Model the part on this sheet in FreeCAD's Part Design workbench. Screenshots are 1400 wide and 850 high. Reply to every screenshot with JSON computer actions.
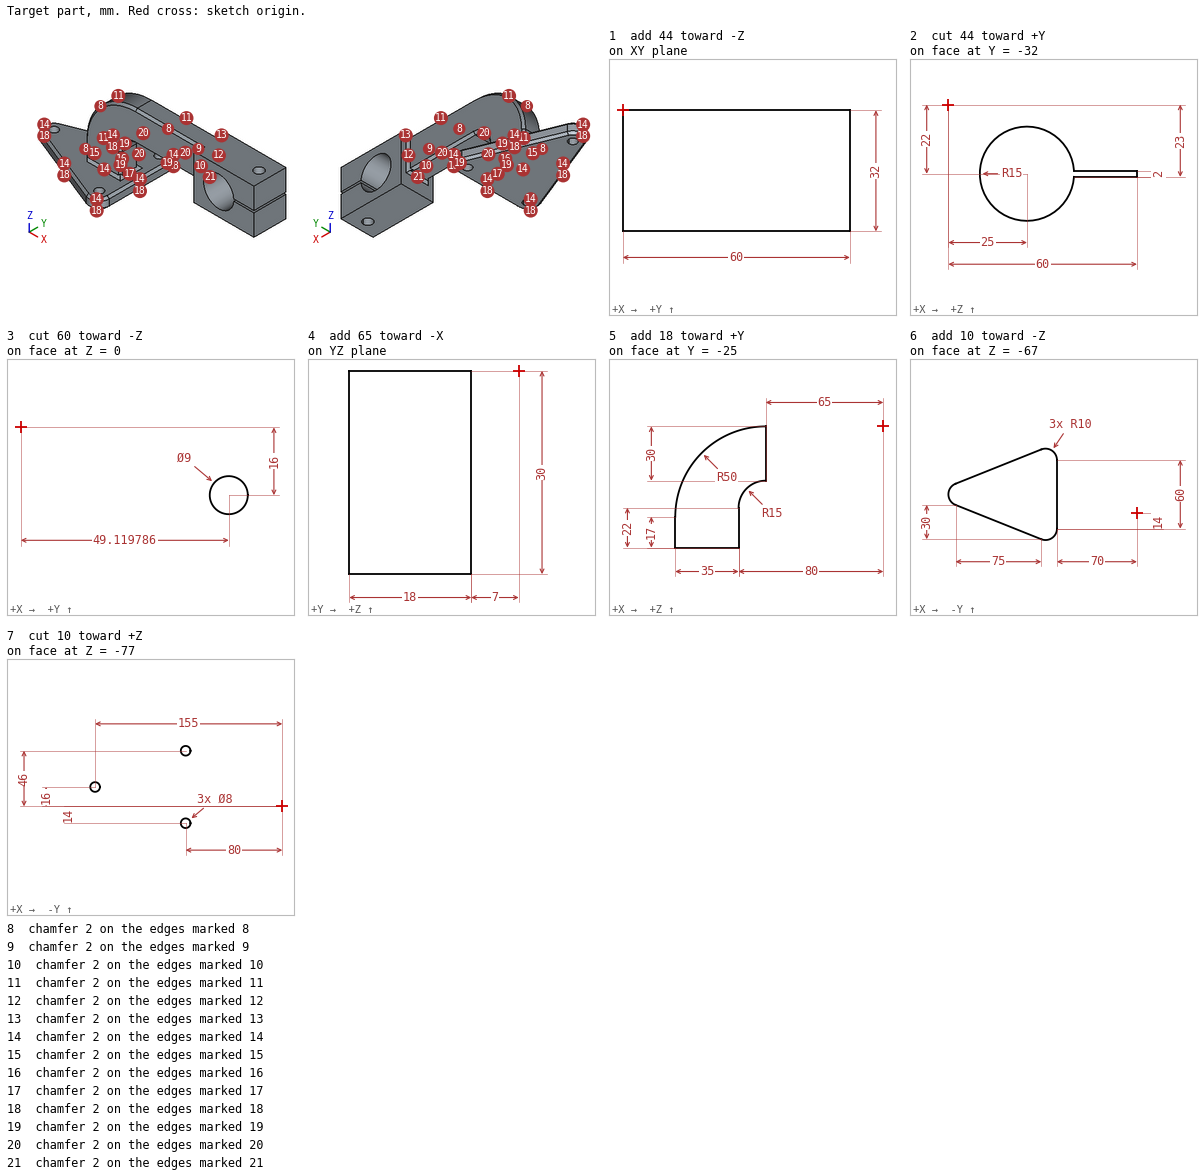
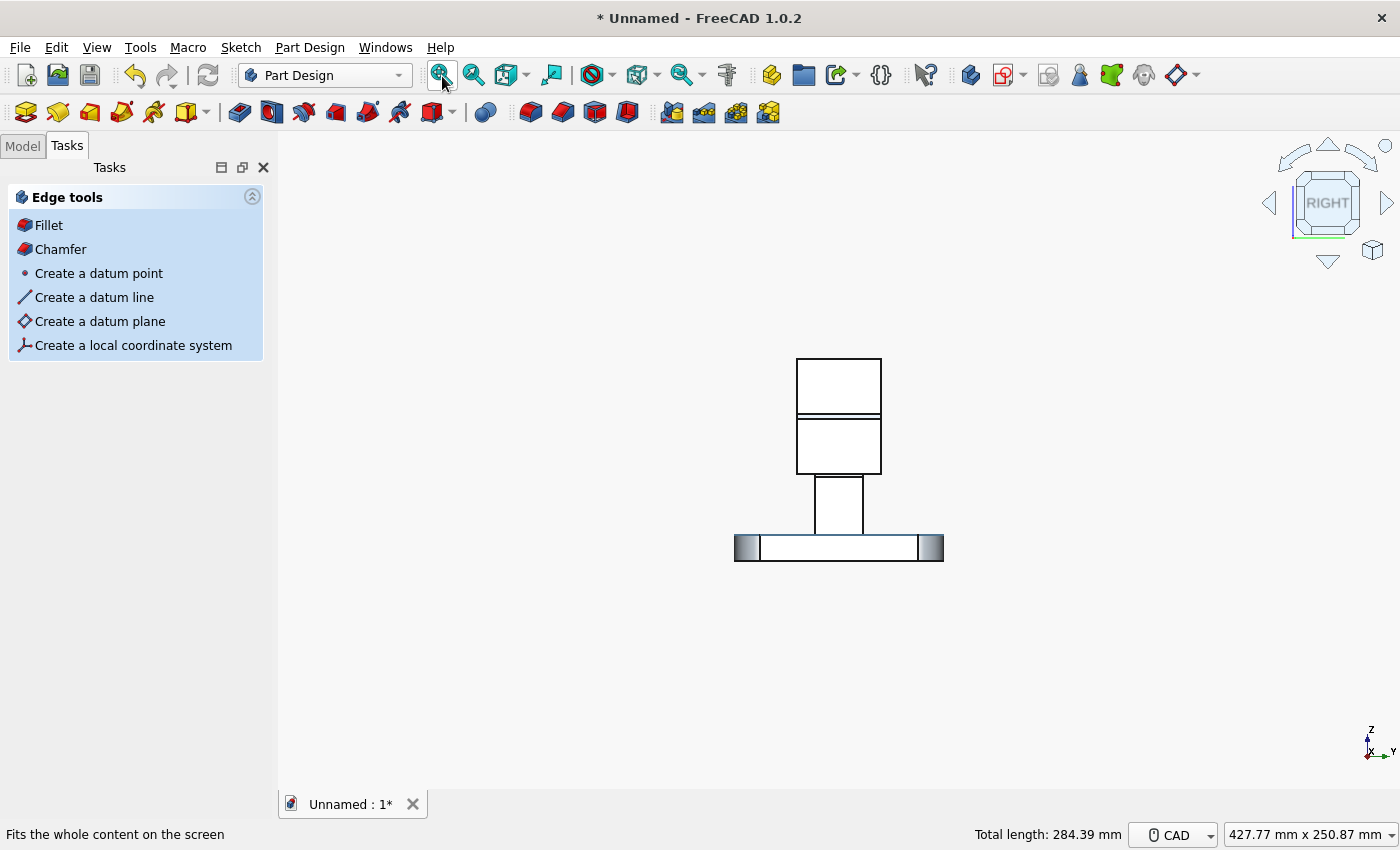
{"action": "key", "text": "5"}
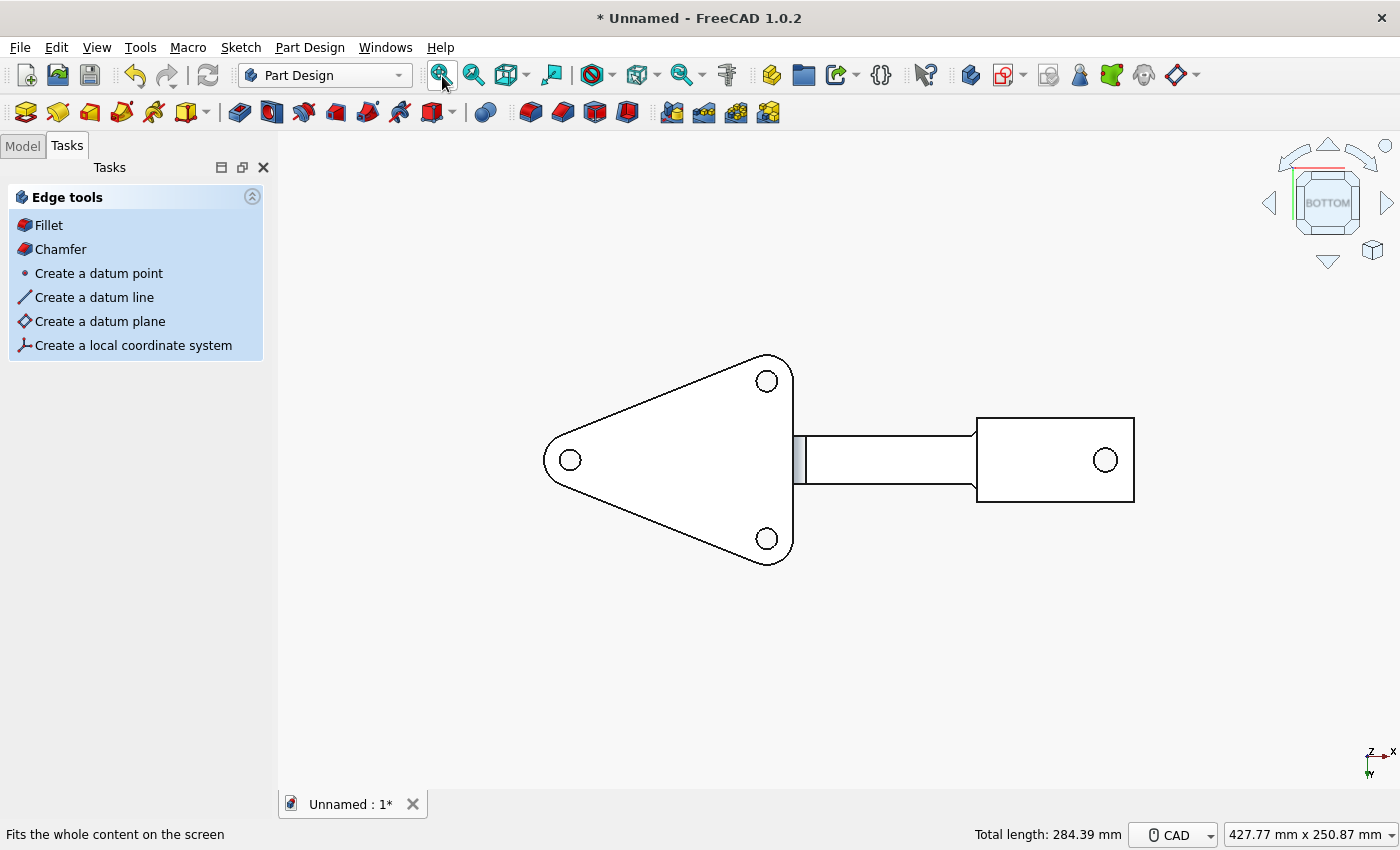
{"action": "key", "text": "4"}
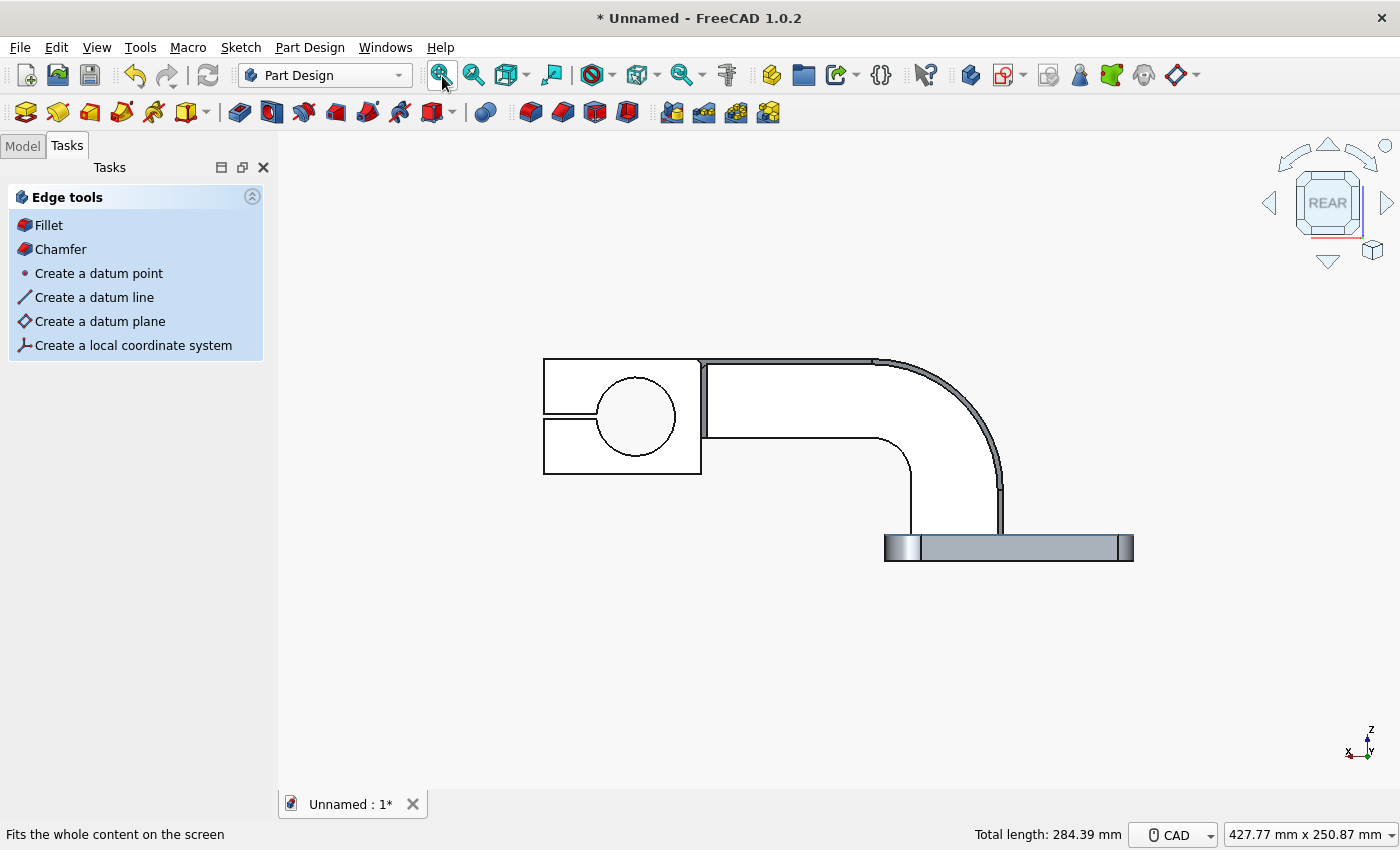
{"action": "key", "text": "6"}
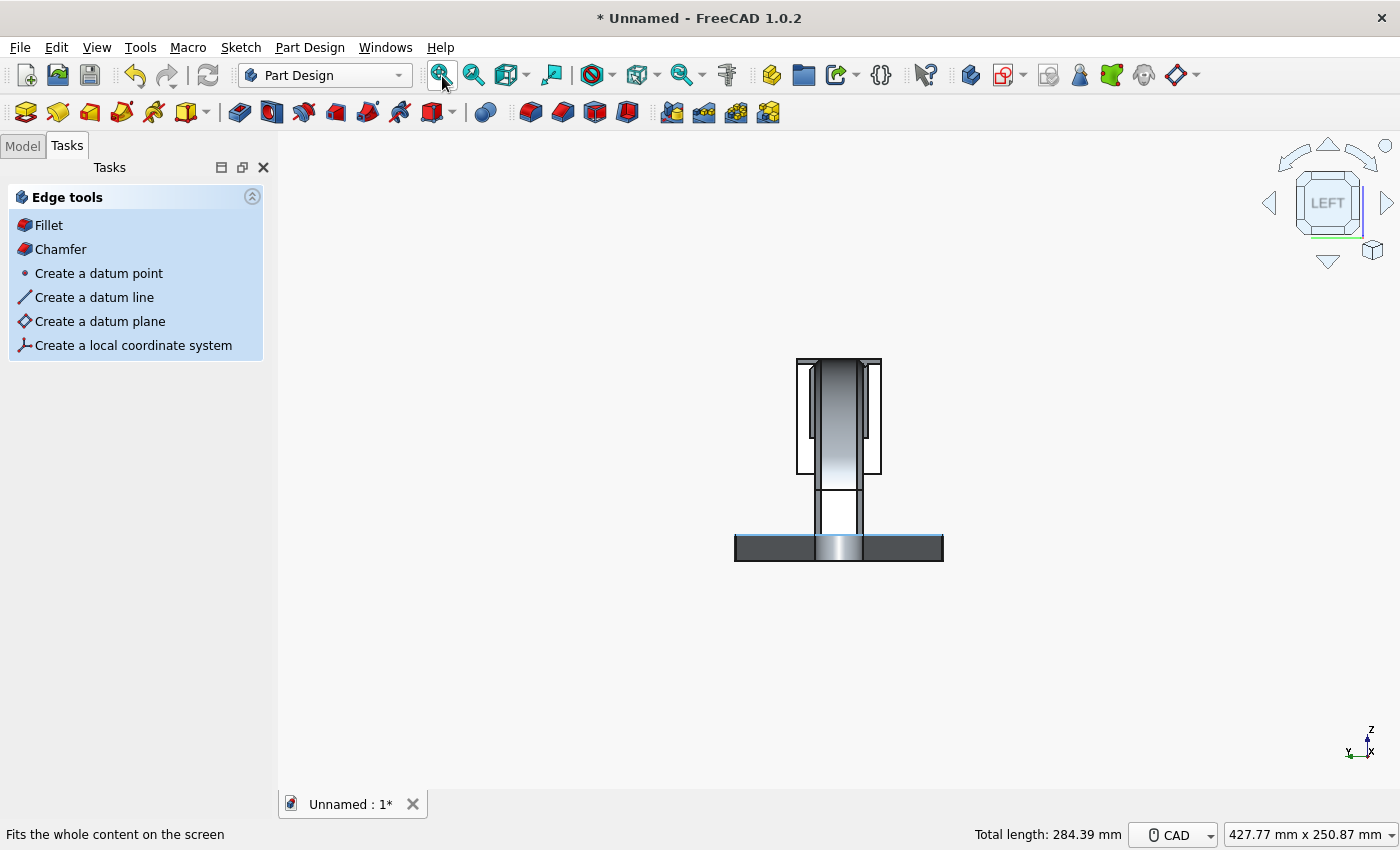
{"action": "key", "text": "v f"}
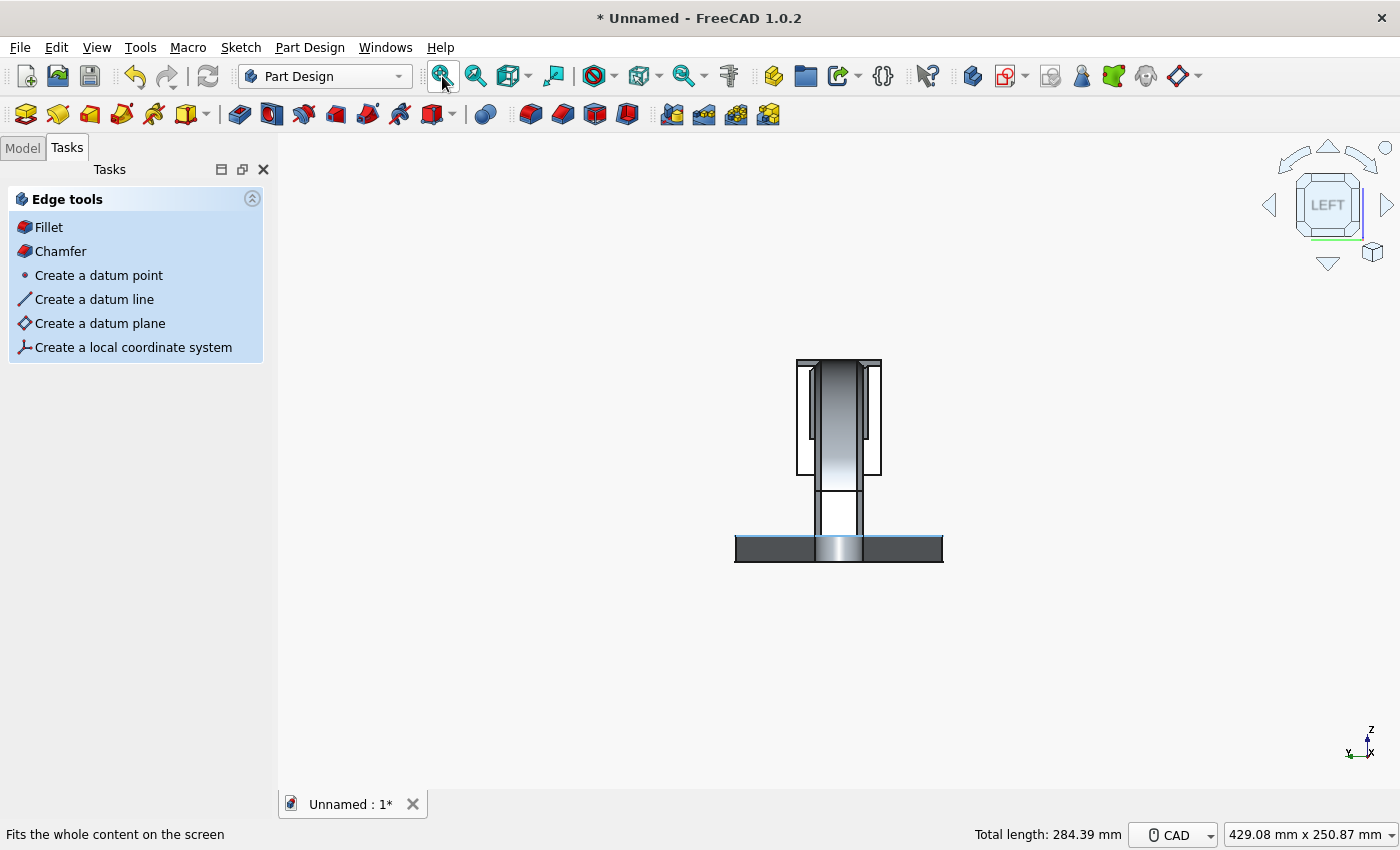
{"action": "key", "text": "v 3"}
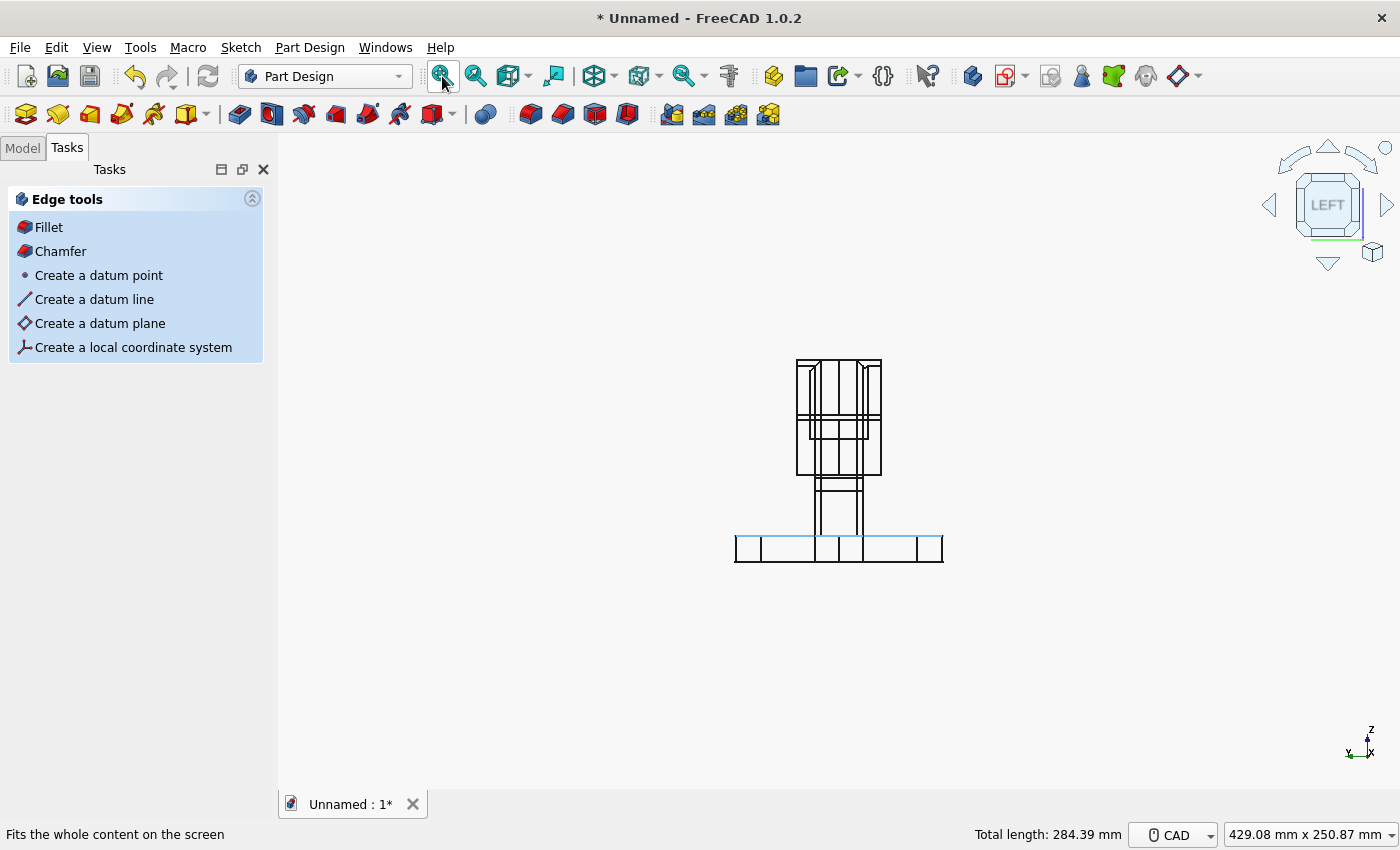
{"action": "key", "text": "0"}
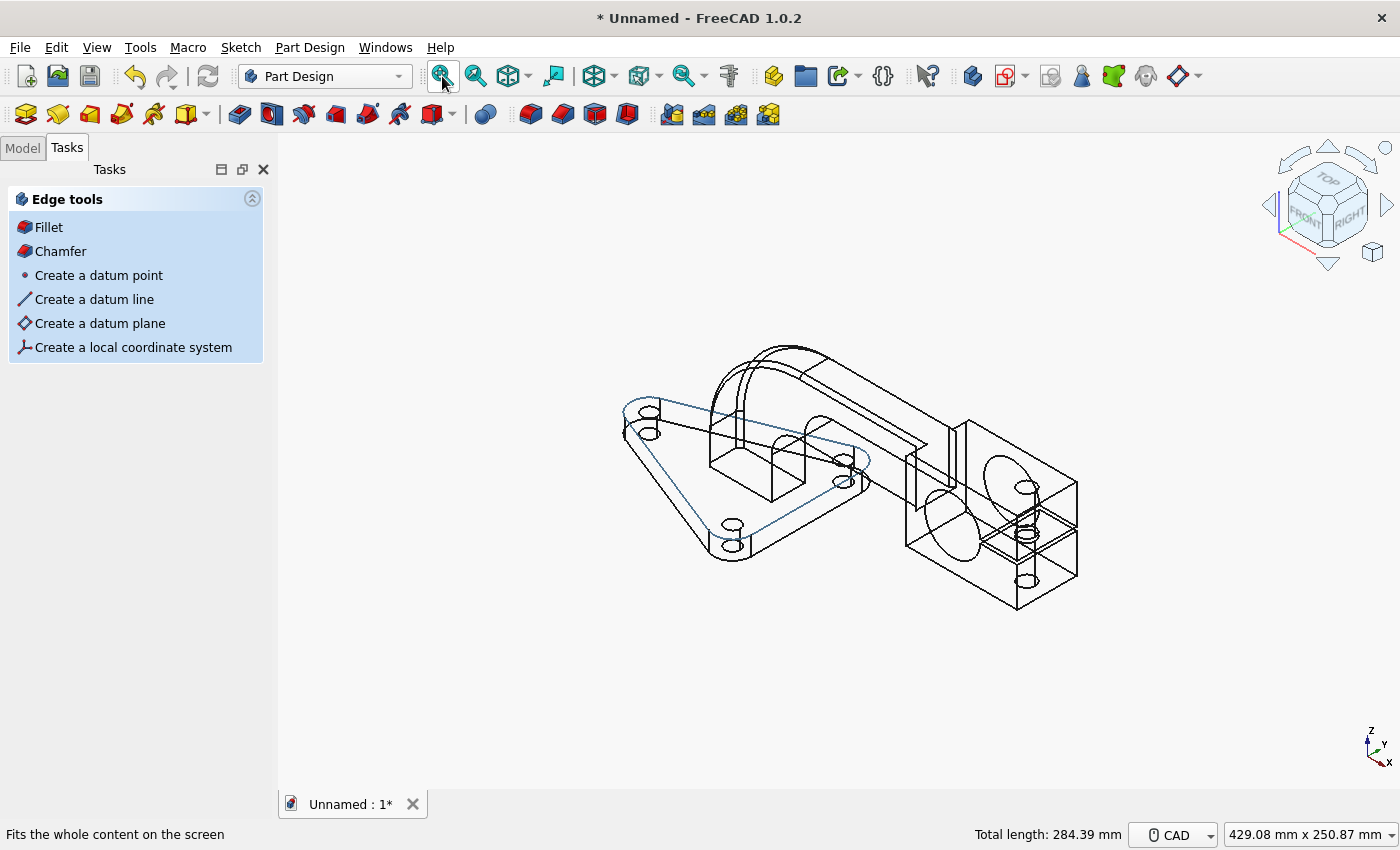
{"action": "left_click", "coordinate": [741, 483], "text": "ctrl"}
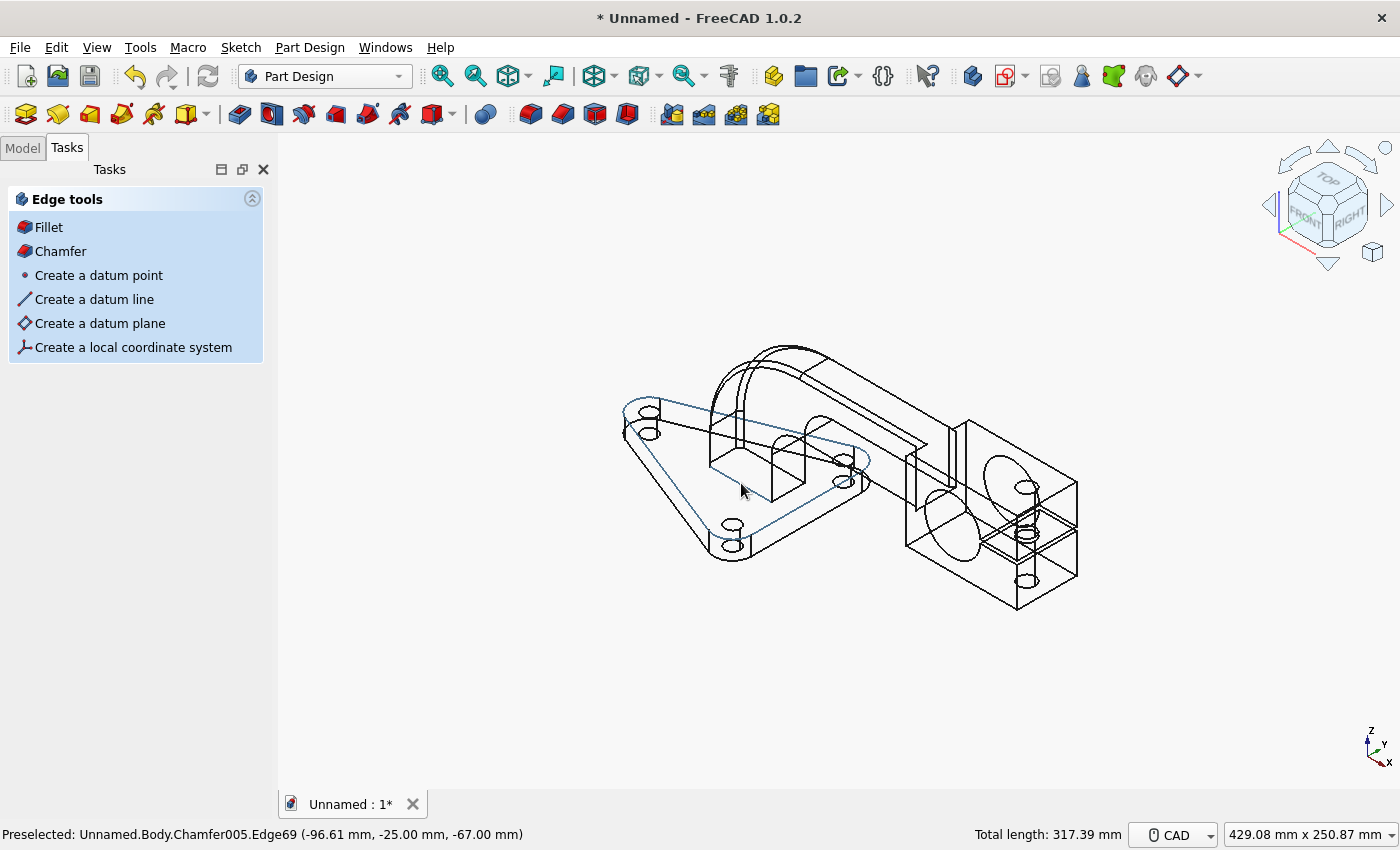
{"action": "key", "text": "v 1"}